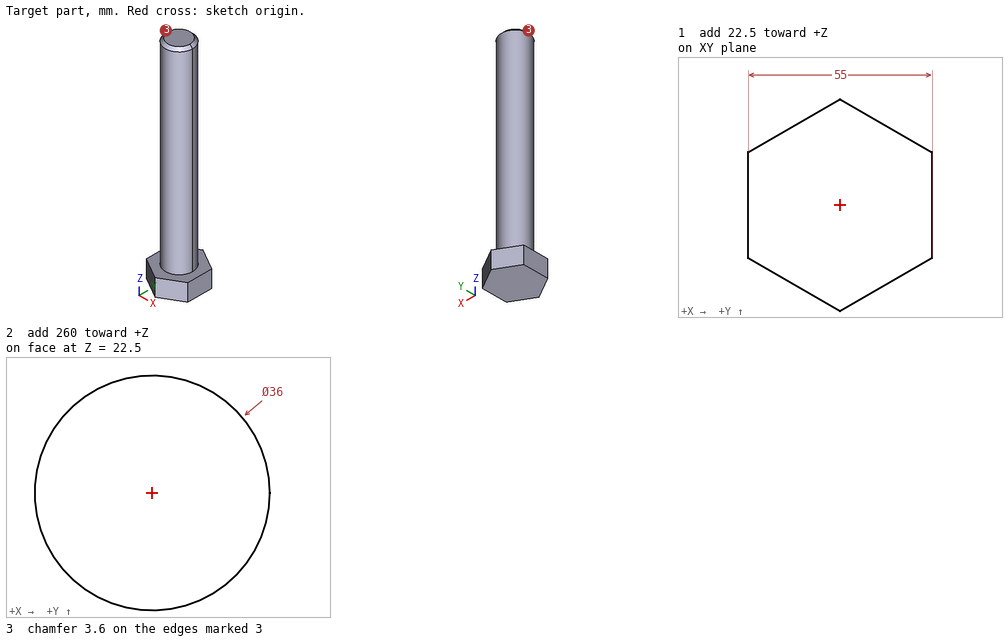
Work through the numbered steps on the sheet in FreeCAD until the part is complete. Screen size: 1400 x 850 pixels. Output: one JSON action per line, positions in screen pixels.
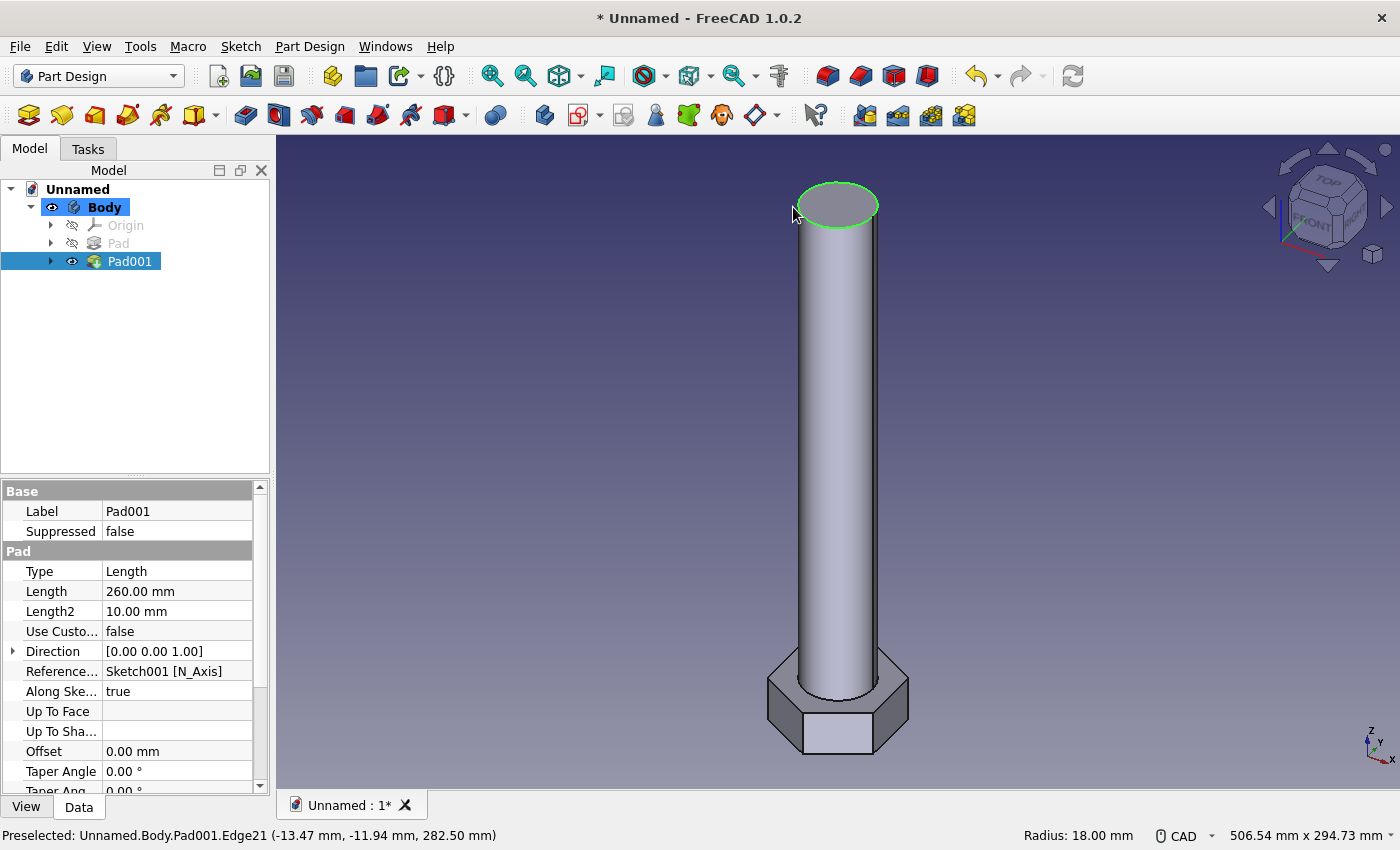
{"action": "left_click", "coordinate": [861, 76]}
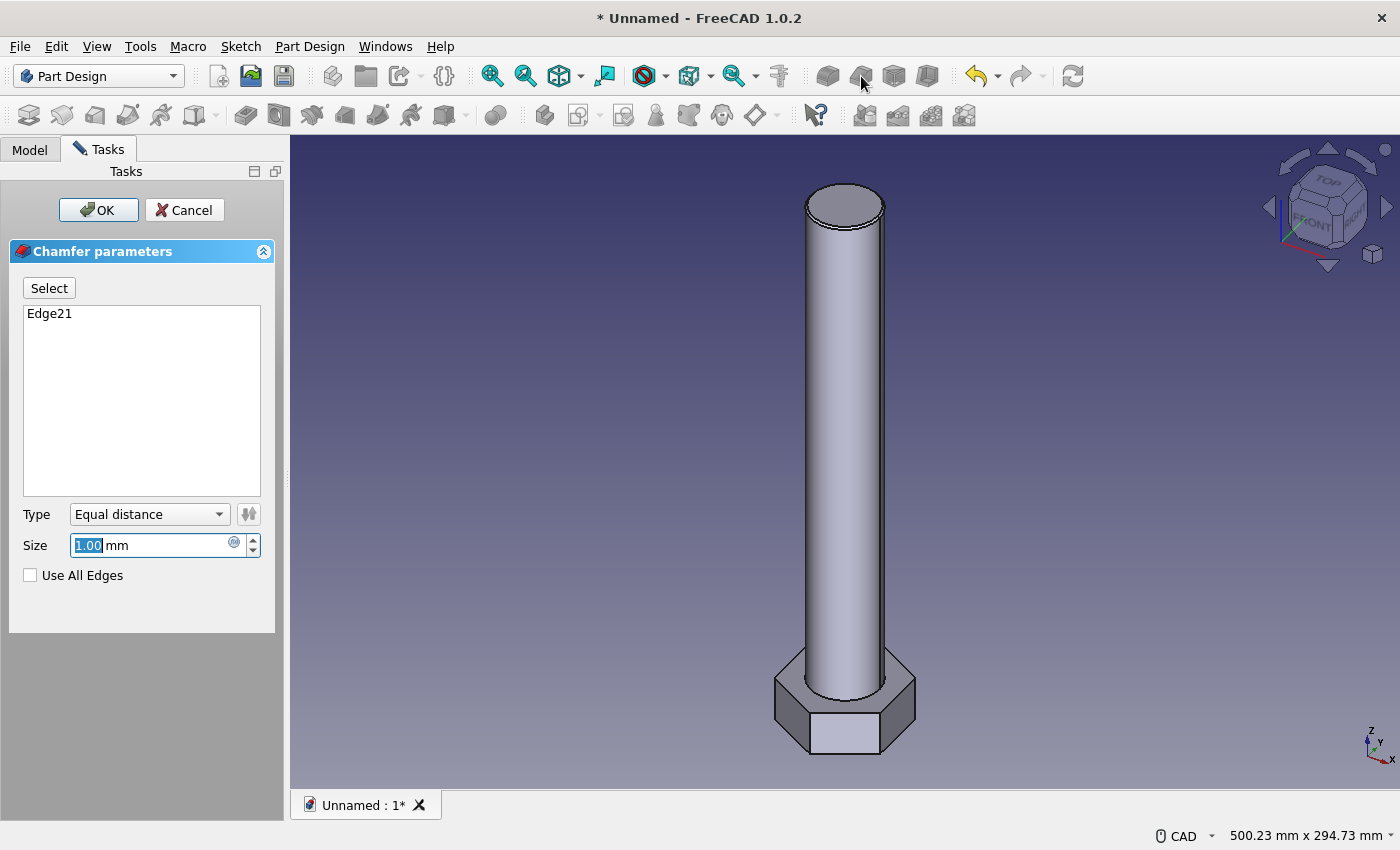
{"action": "type", "text": "3.6"}
{"action": "key", "text": "Tab"}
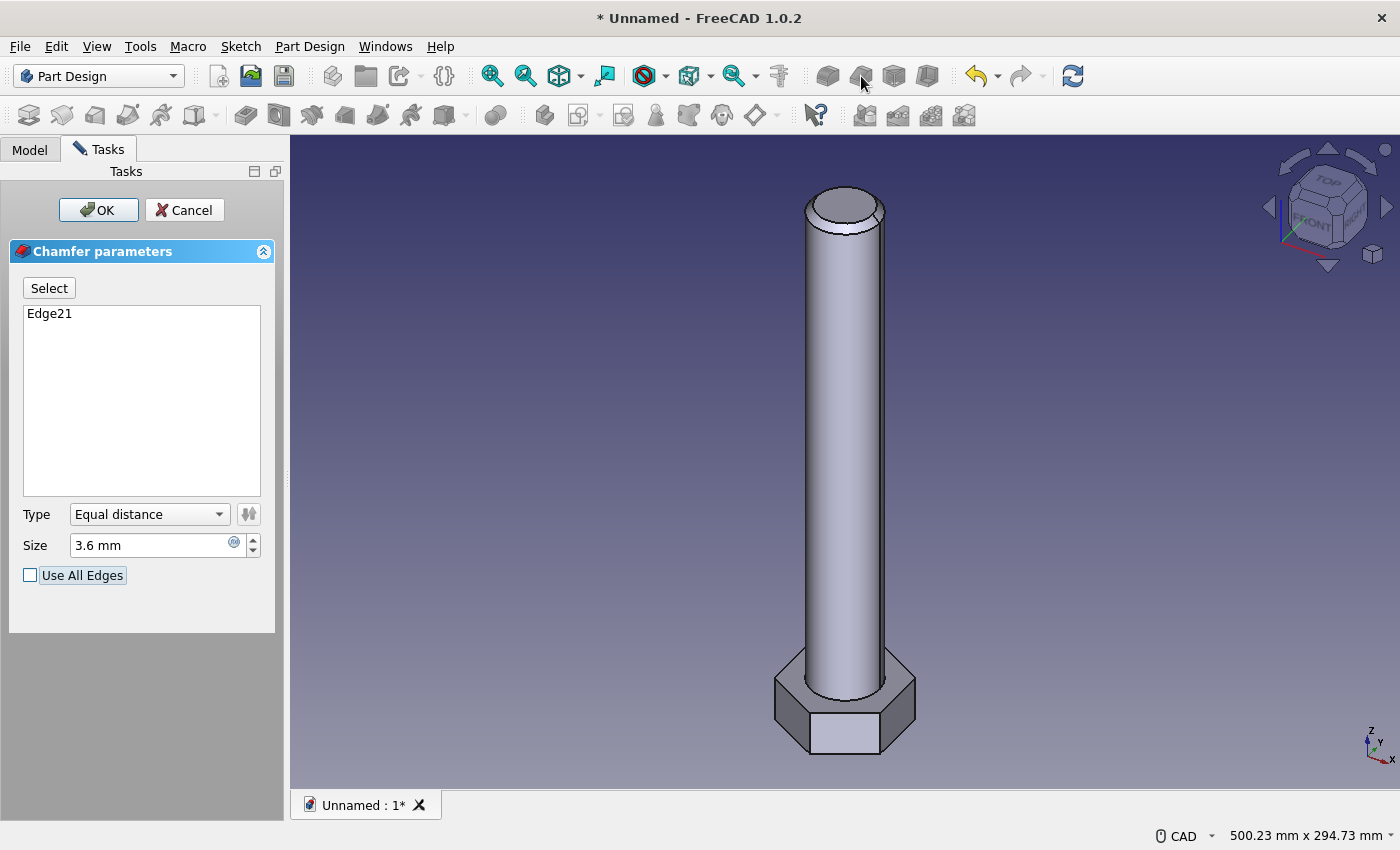
{"action": "left_click", "coordinate": [99, 210]}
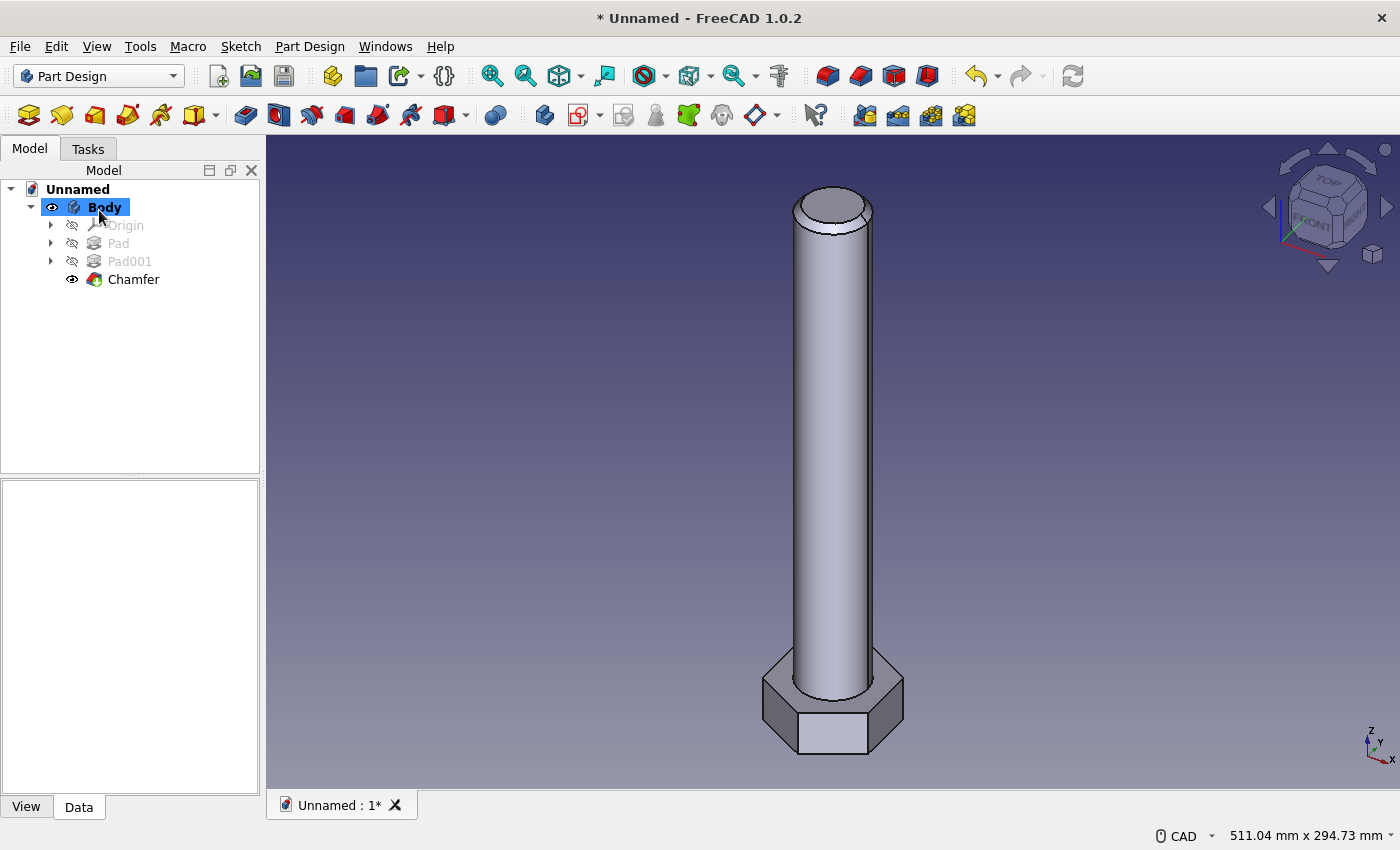
{"action": "key", "text": "0"}